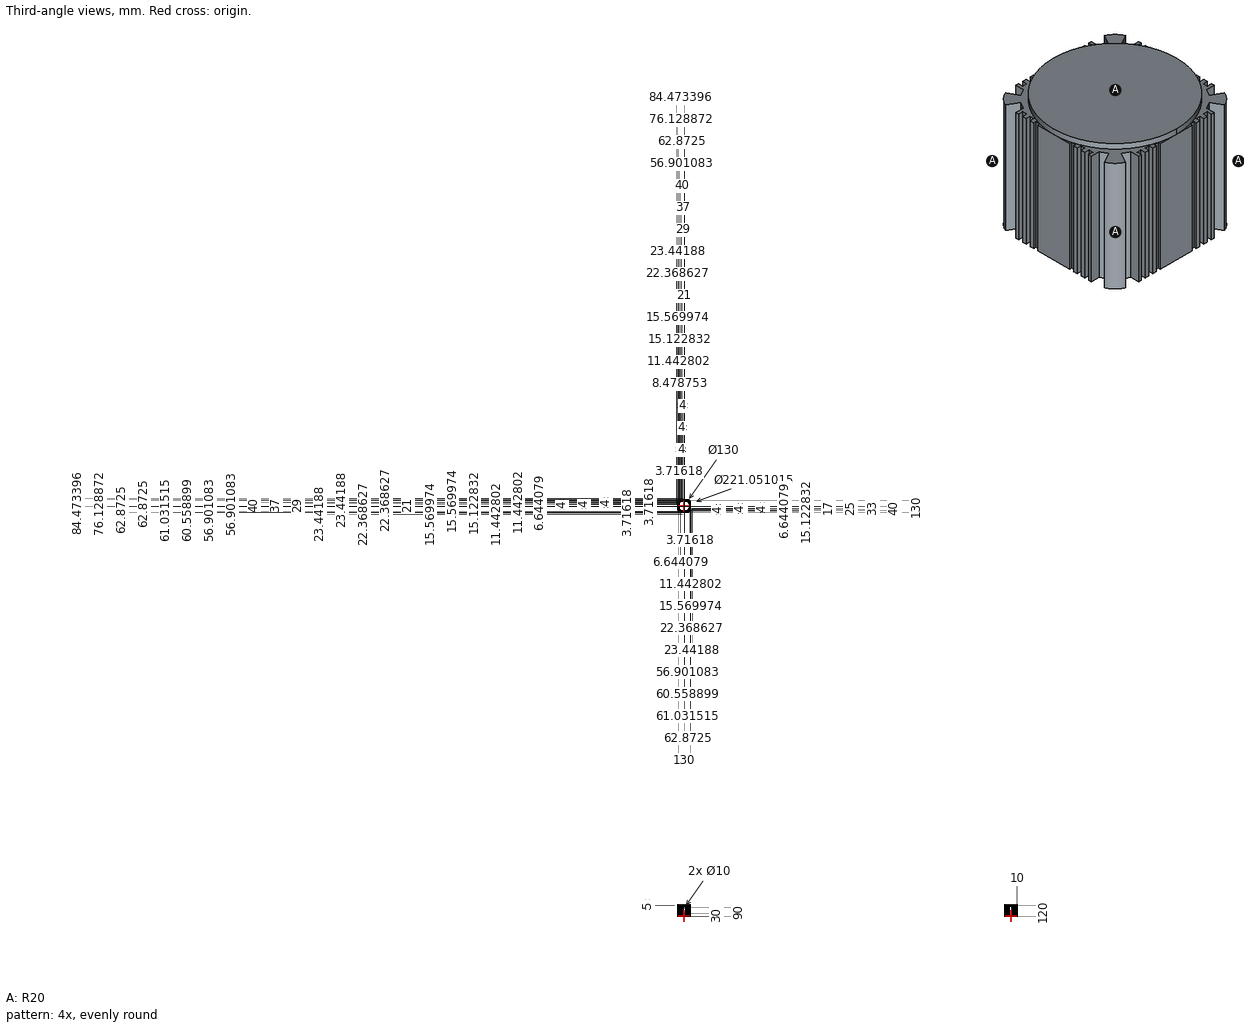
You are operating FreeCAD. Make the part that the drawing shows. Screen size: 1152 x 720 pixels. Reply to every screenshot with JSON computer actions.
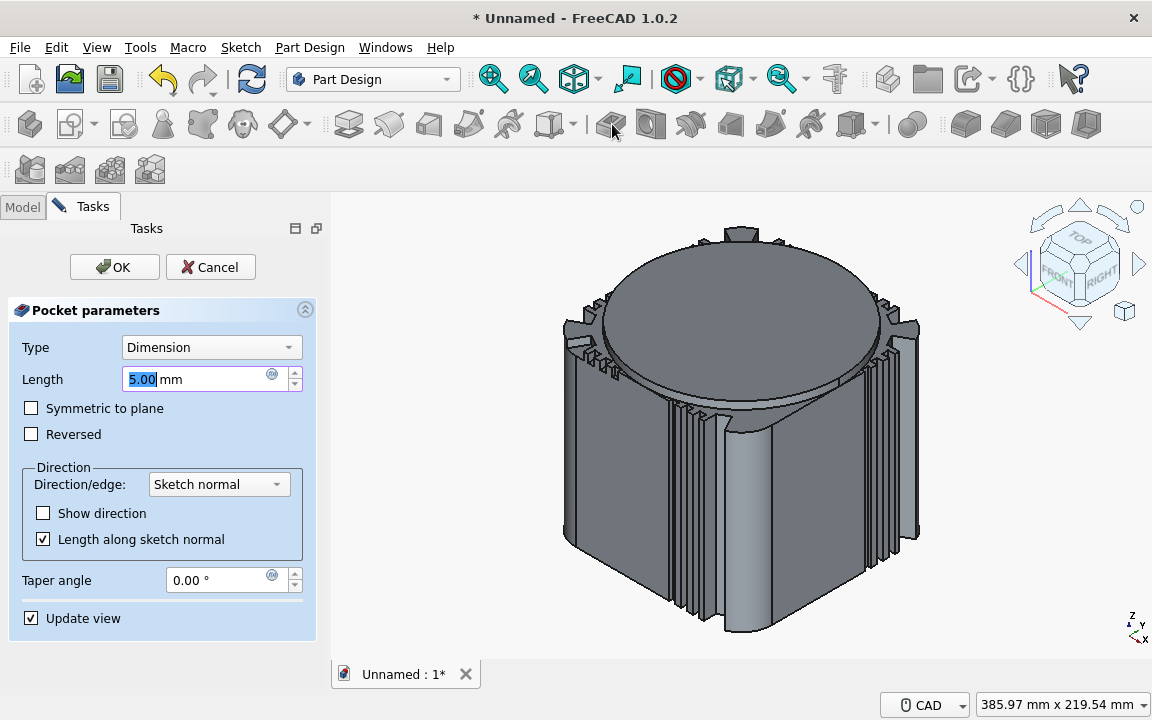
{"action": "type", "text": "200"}
{"action": "key", "text": "Tab"}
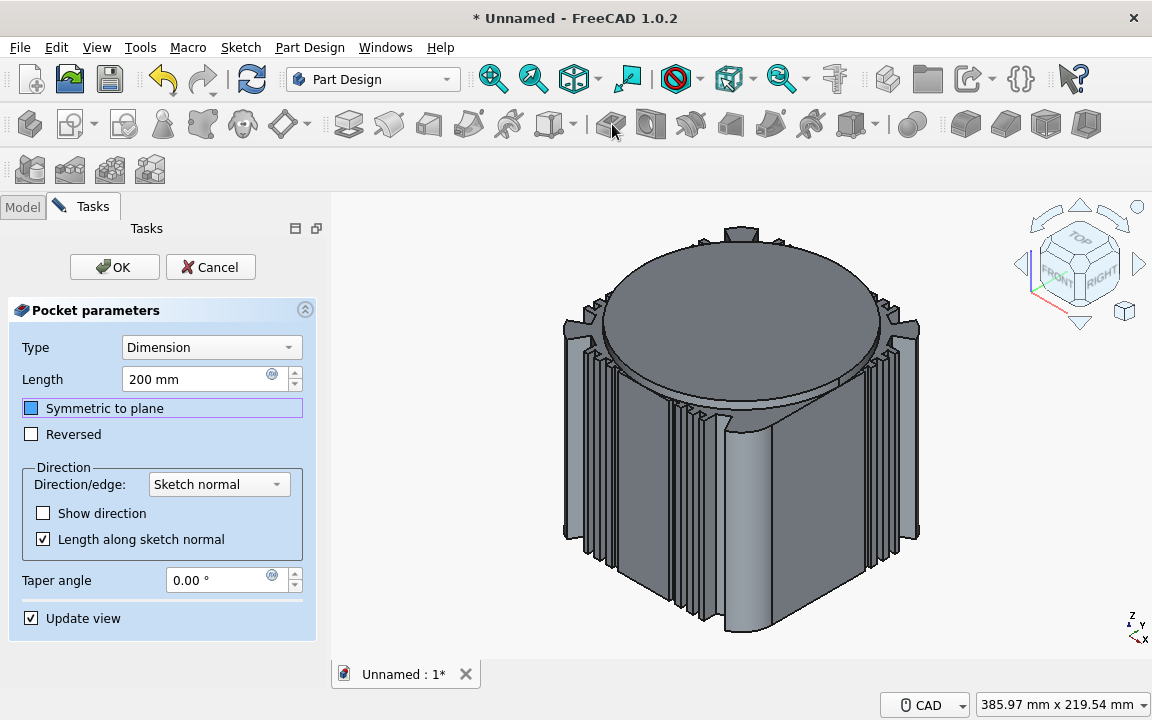
{"action": "left_click", "coordinate": [115, 267]}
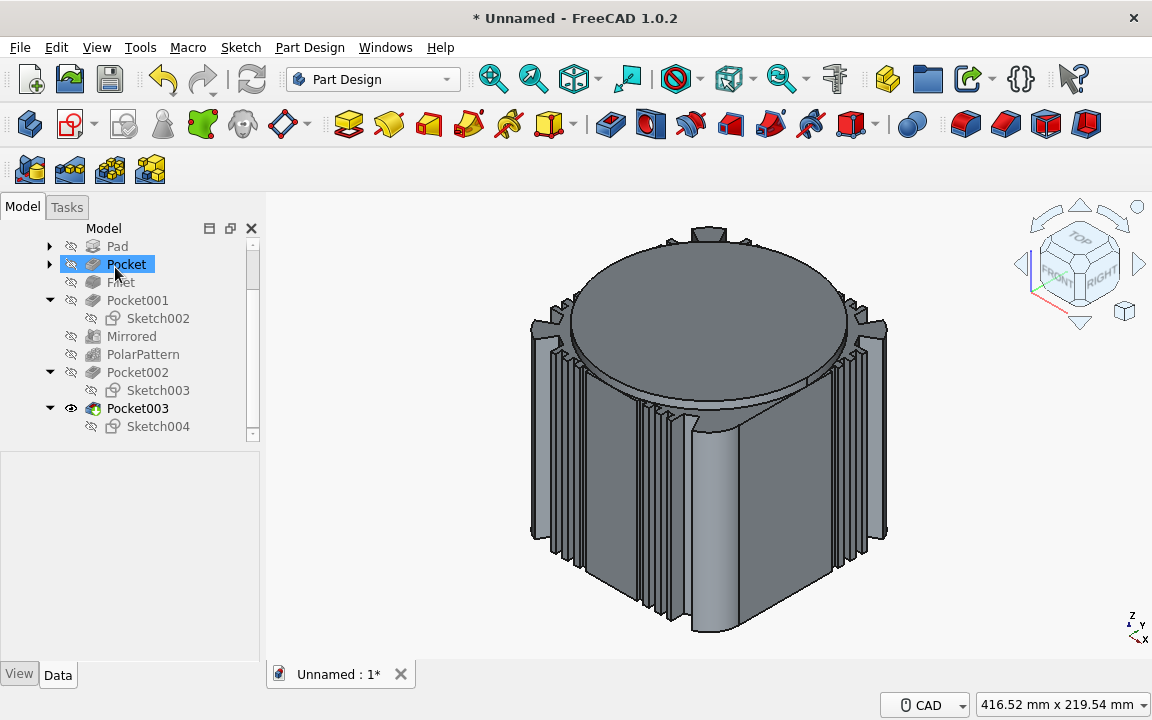
{"action": "left_click", "coordinate": [709, 418]}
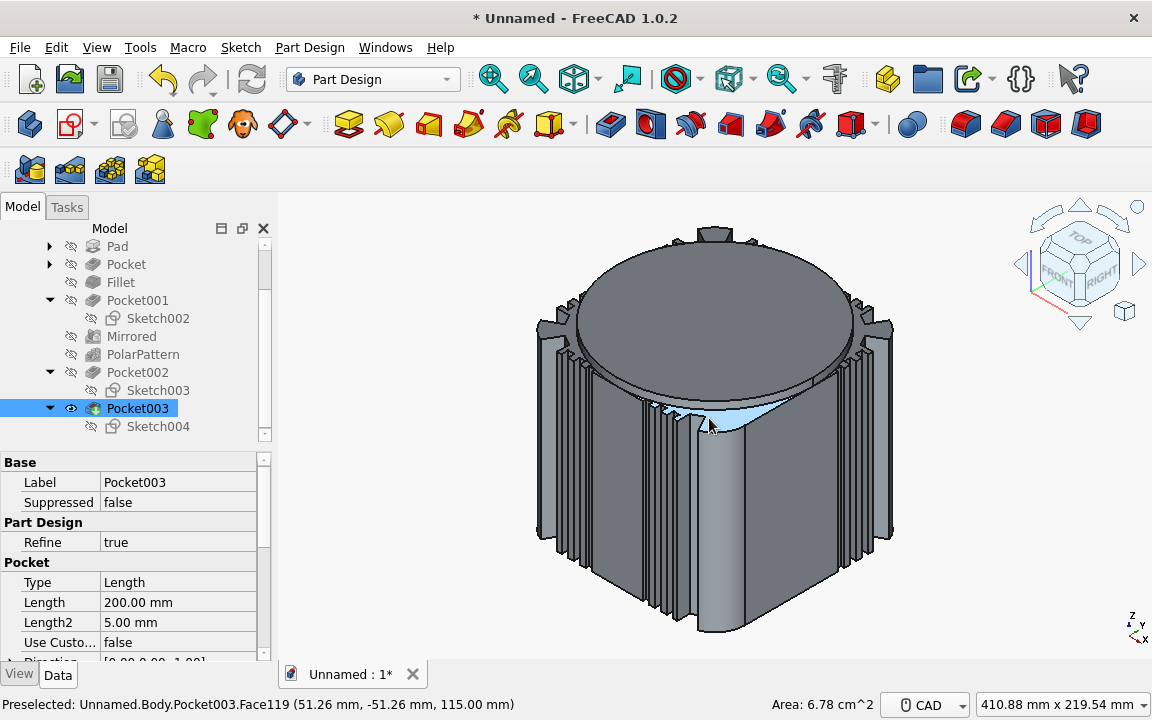
{"action": "left_click", "coordinate": [70, 124]}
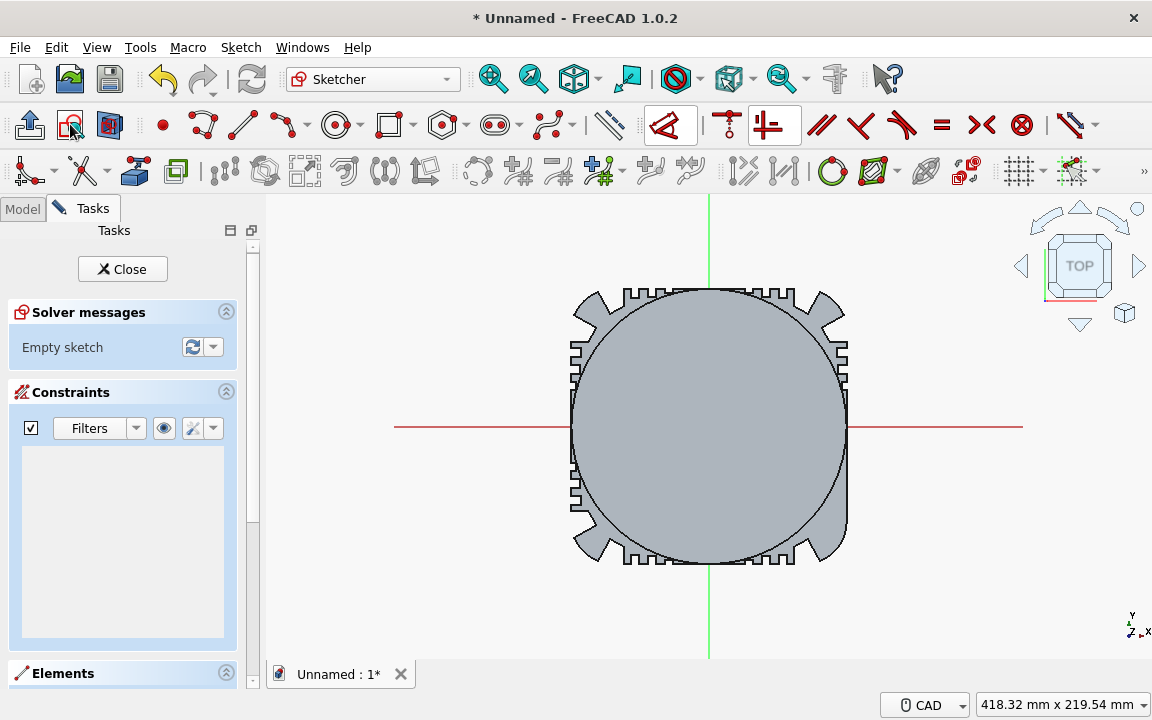
{"action": "scroll", "coordinate": [892, 519], "scroll_direction": "up", "scroll_amount": 5}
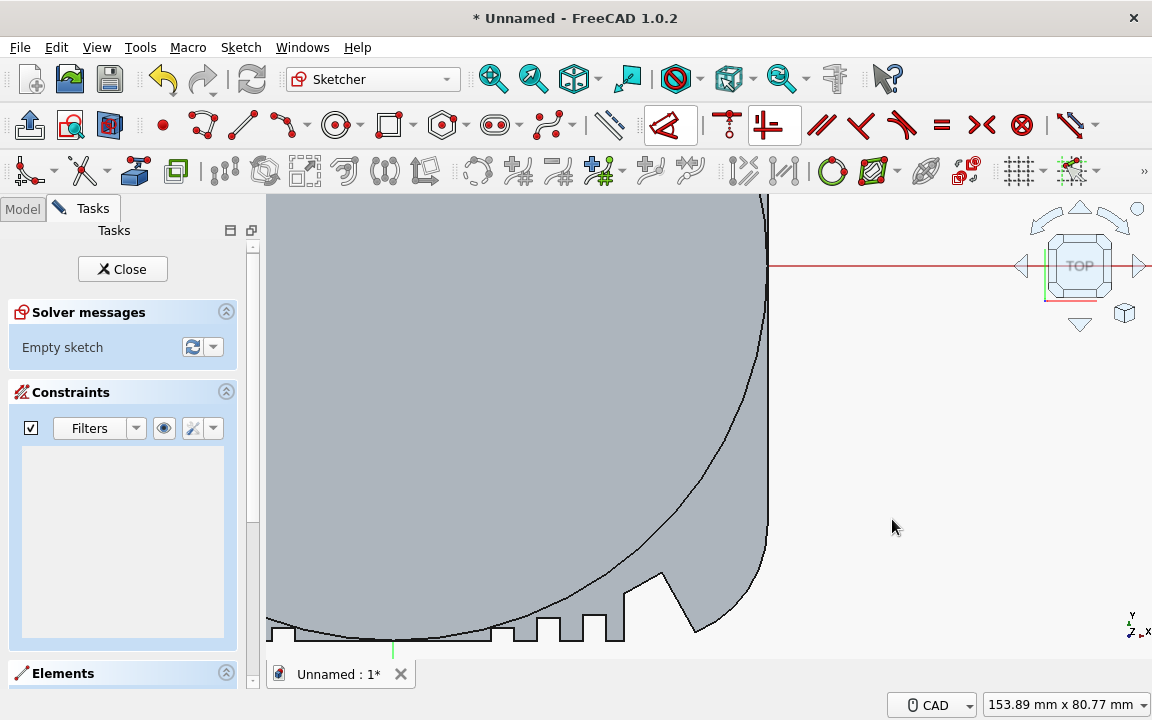
{"action": "left_click", "coordinate": [204, 126]}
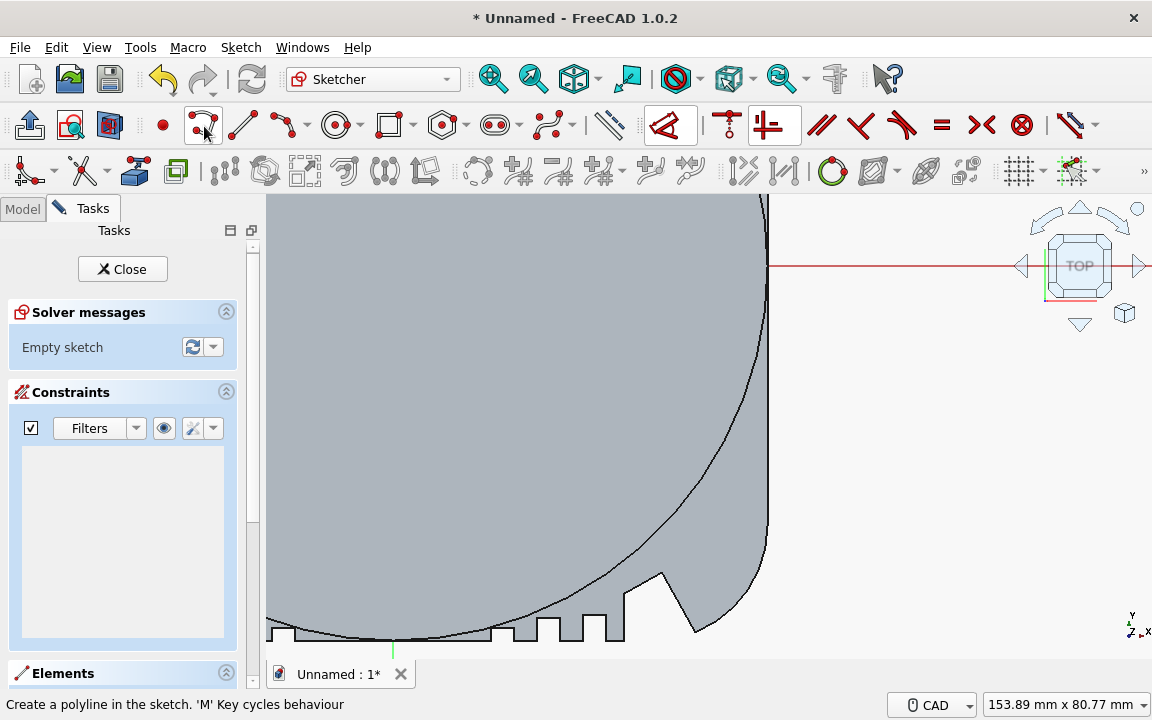
{"action": "left_click", "coordinate": [721, 497]}
{"action": "left_click", "coordinate": [700, 535]}
{"action": "left_click", "coordinate": [787, 584]}
{"action": "left_click", "coordinate": [787, 497]}
{"action": "left_click", "coordinate": [721, 498]}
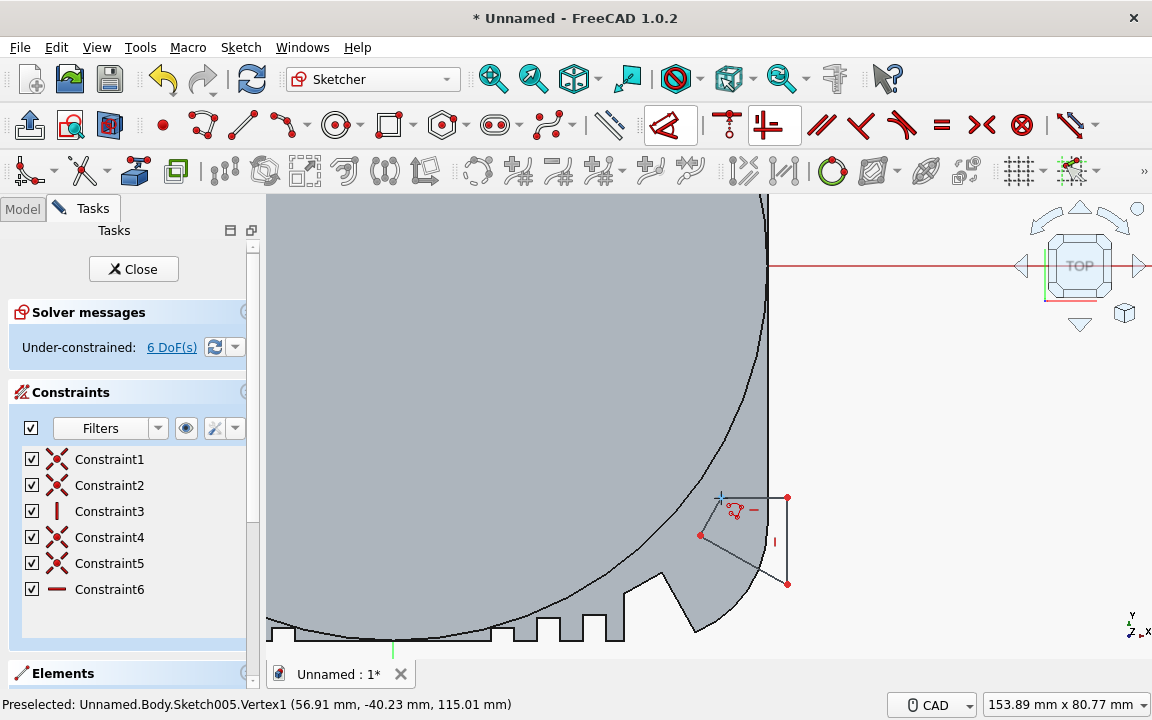
{"action": "key", "text": "g r"}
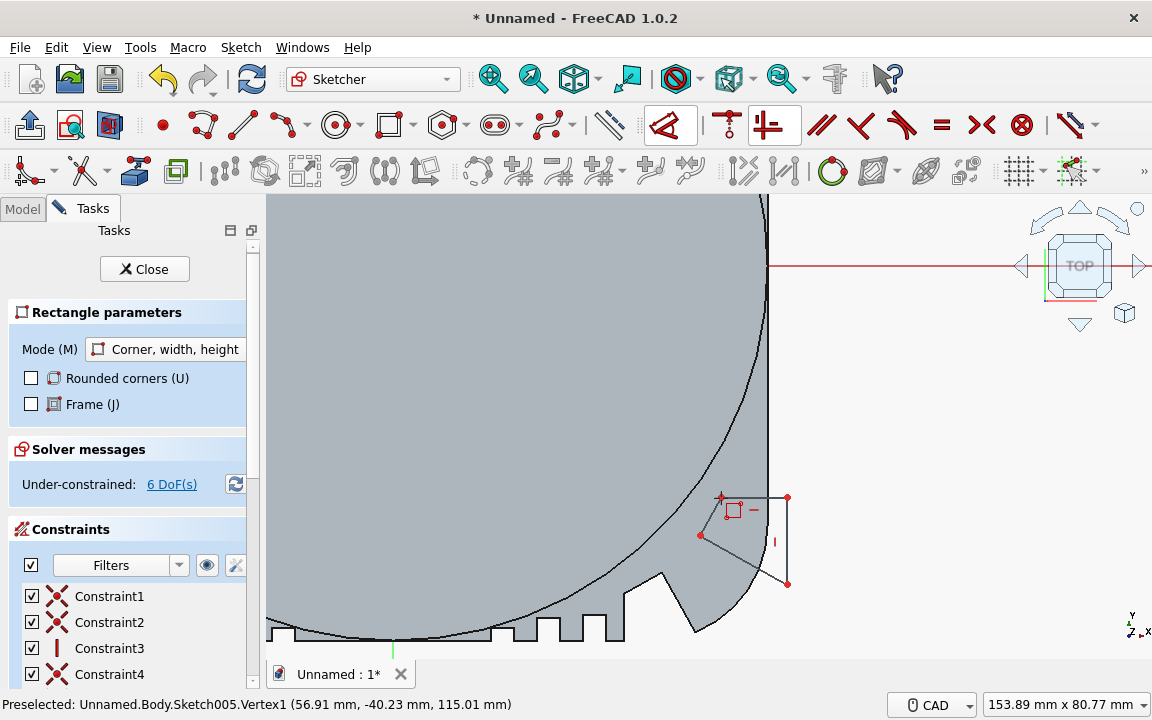
{"action": "left_click", "coordinate": [742, 456]}
{"action": "mouse_move", "coordinate": [832, 479]}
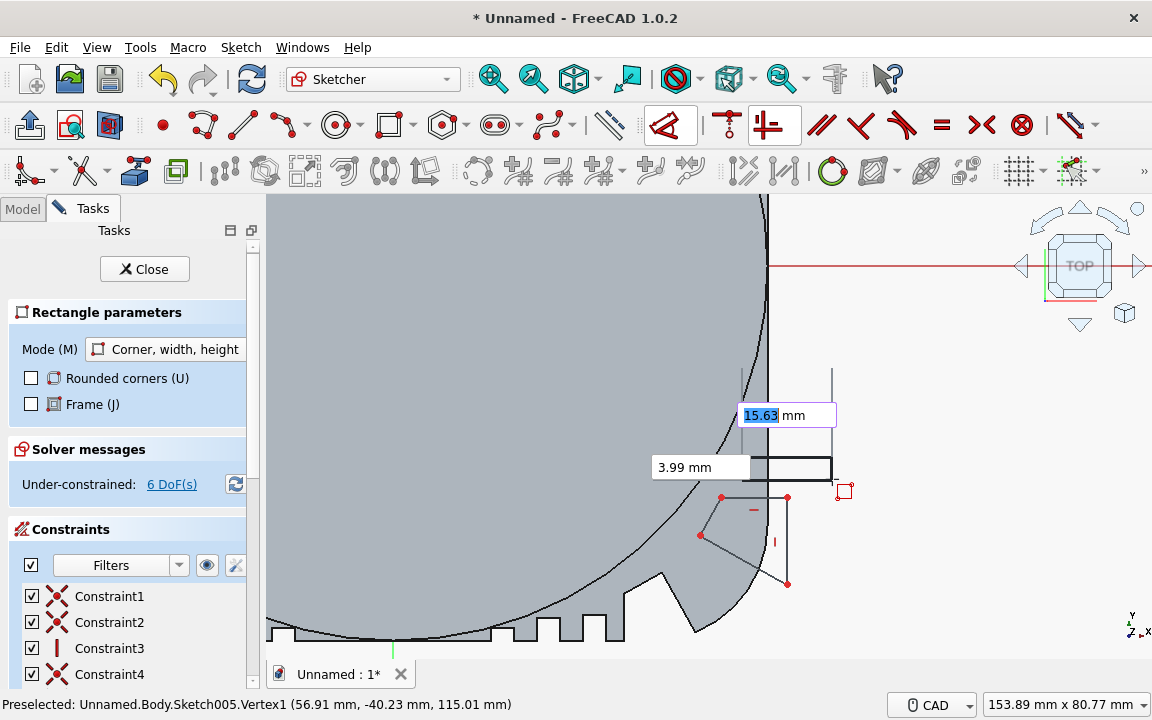
{"action": "type", "text": "15.569974"}
{"action": "key", "text": "Tab"}
{"action": "type", "text": "4"}
{"action": "key", "text": "Return"}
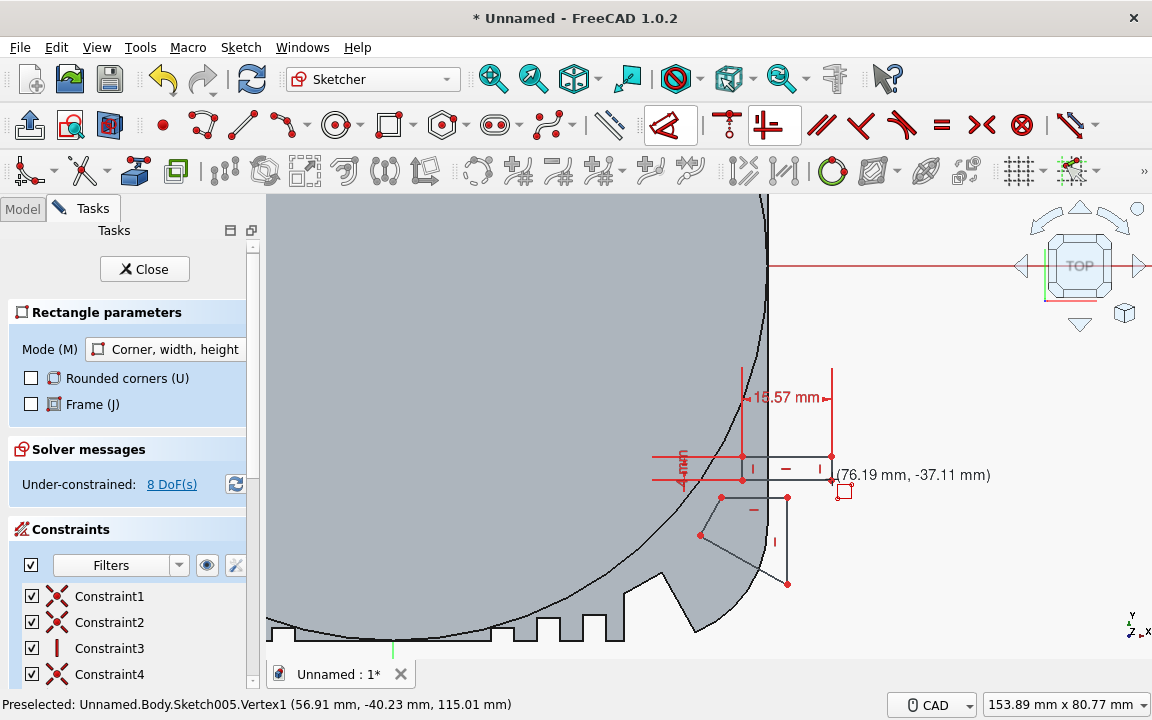
{"action": "left_click", "coordinate": [745, 410]}
{"action": "mouse_move", "coordinate": [880, 433]}